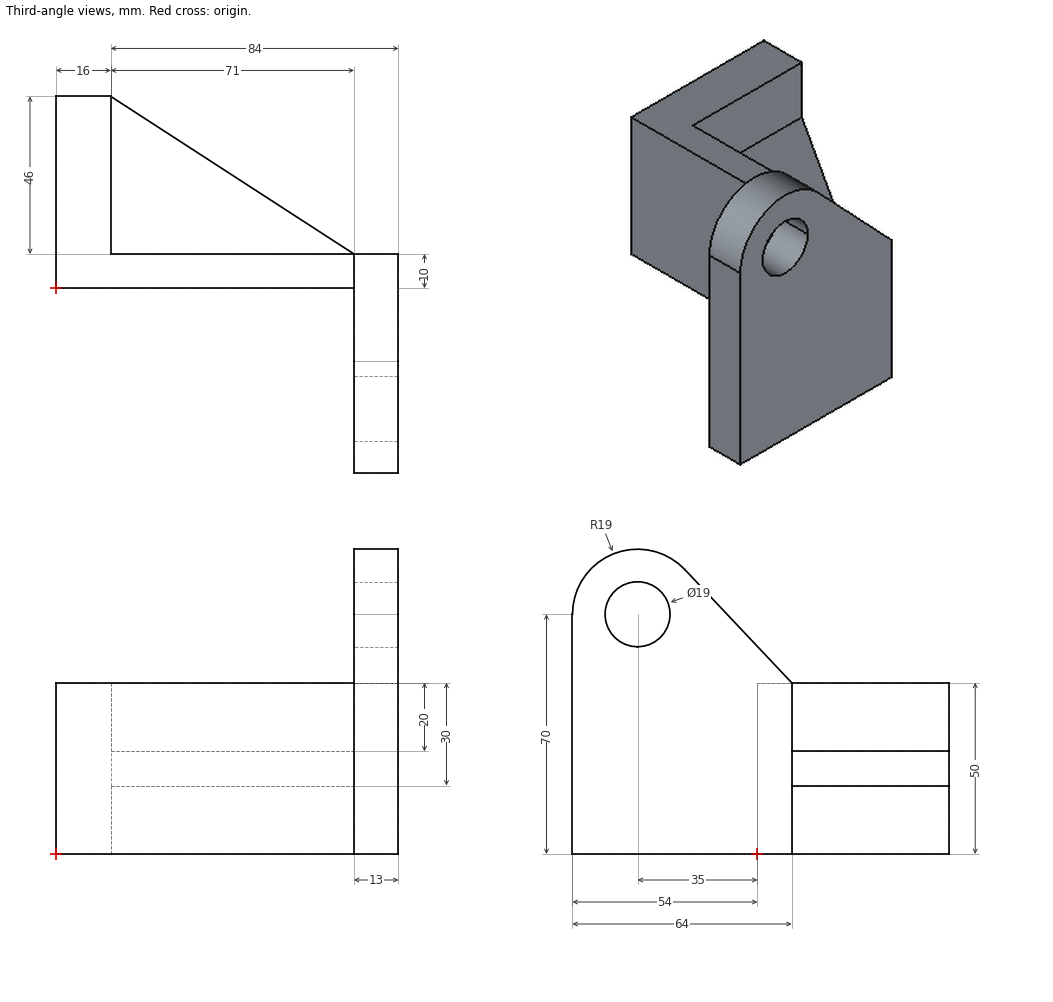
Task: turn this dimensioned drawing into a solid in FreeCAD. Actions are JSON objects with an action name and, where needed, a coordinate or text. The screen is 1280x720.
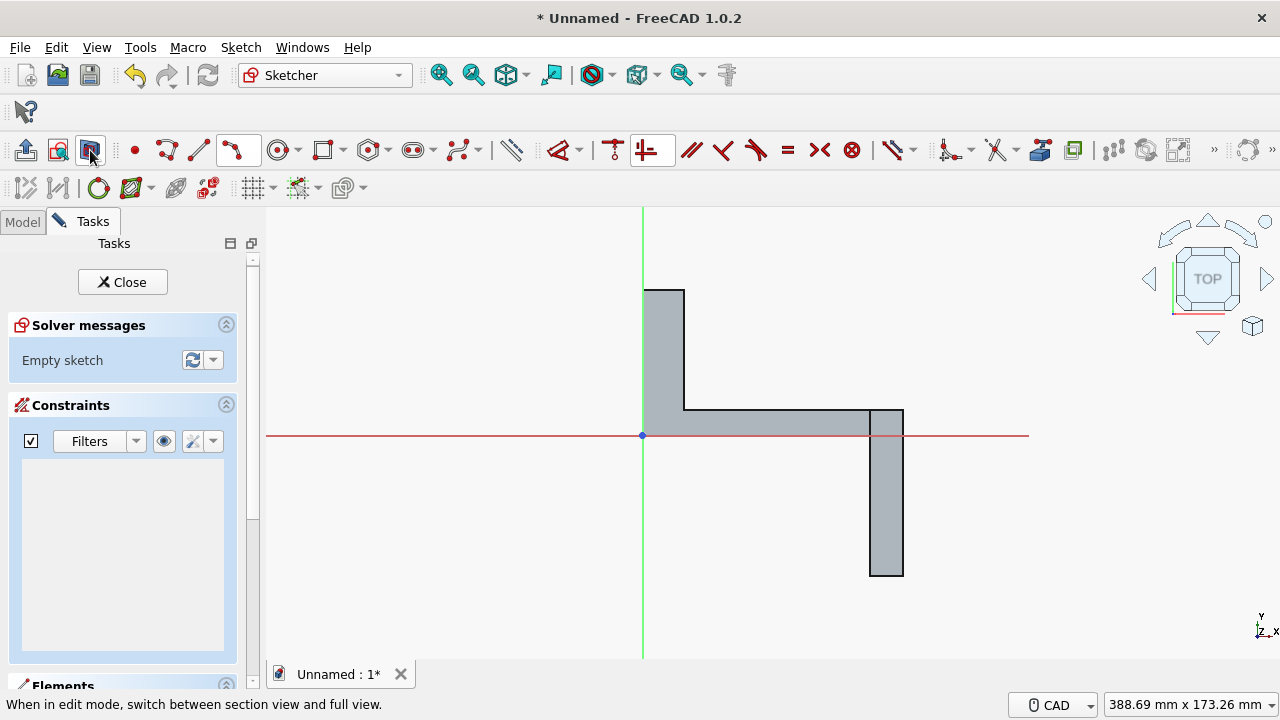
{"action": "scroll", "coordinate": [819, 277], "scroll_direction": "up", "scroll_amount": 3}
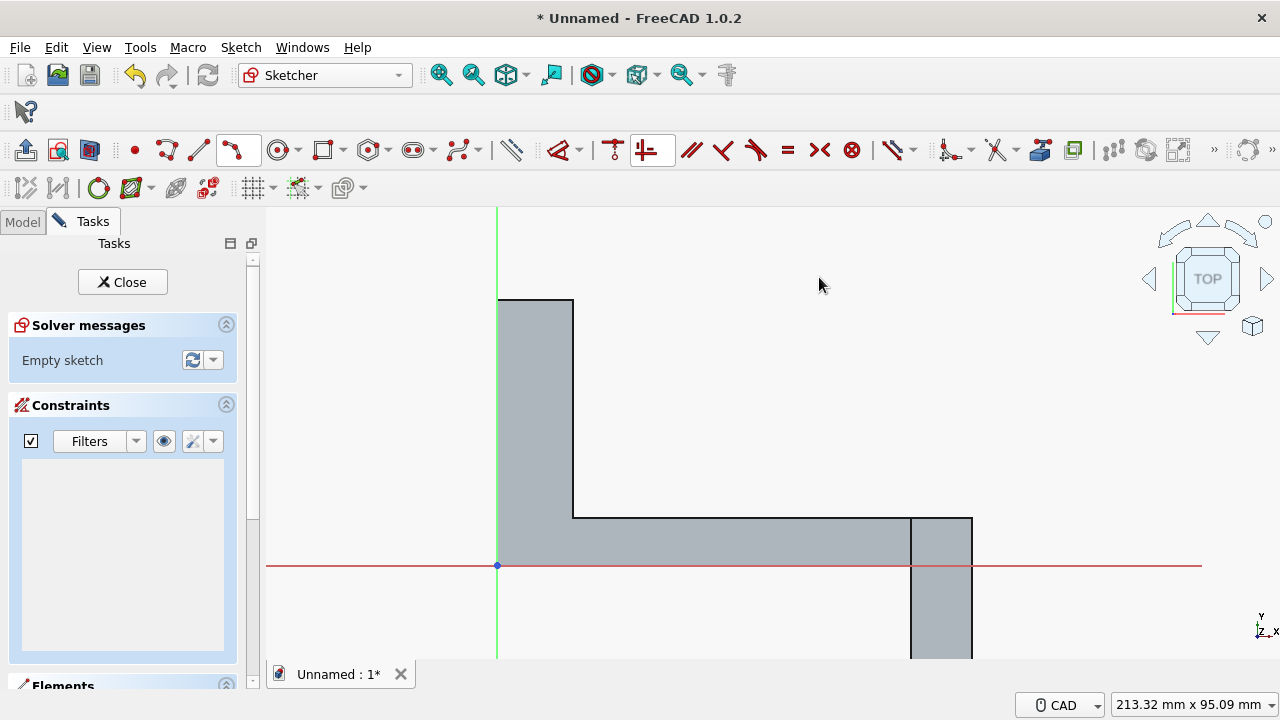
{"action": "left_click", "coordinate": [168, 150]}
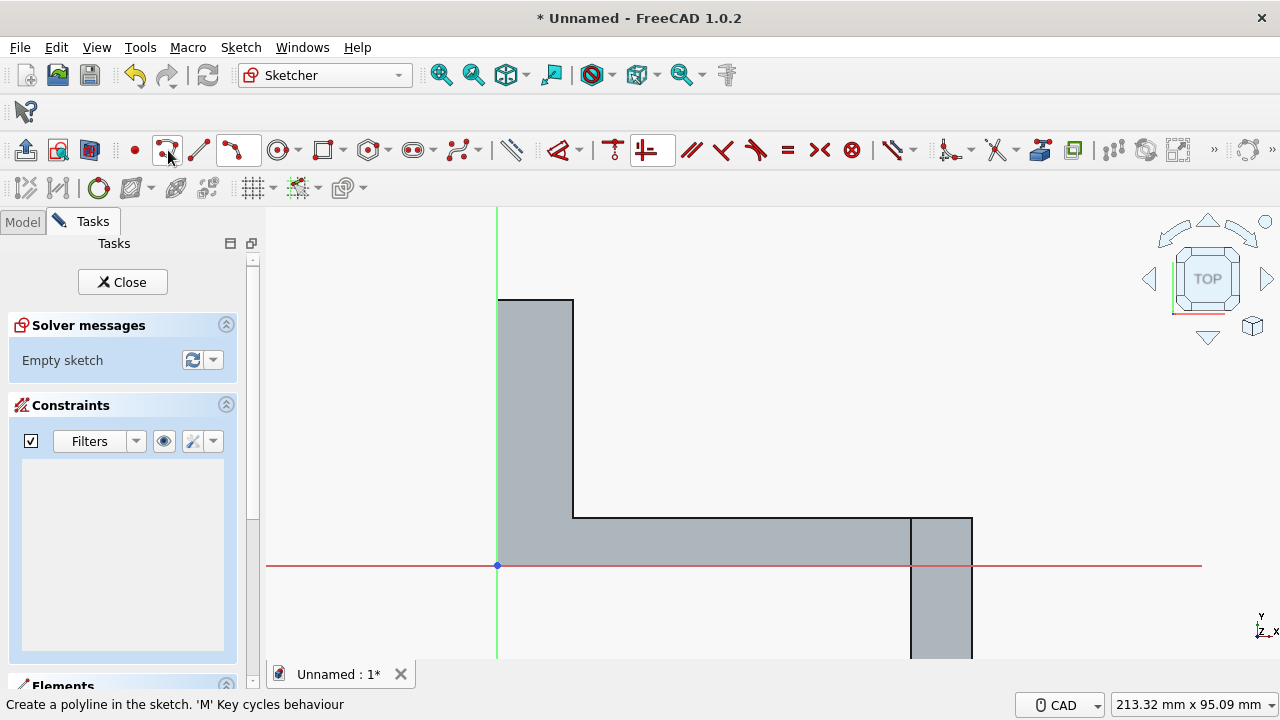
{"action": "left_click", "coordinate": [573, 518]}
{"action": "left_click", "coordinate": [911, 518]}
{"action": "left_click", "coordinate": [573, 300]}
{"action": "left_click", "coordinate": [573, 519]}
{"action": "key", "text": "Escape"}
{"action": "key", "text": "Escape"}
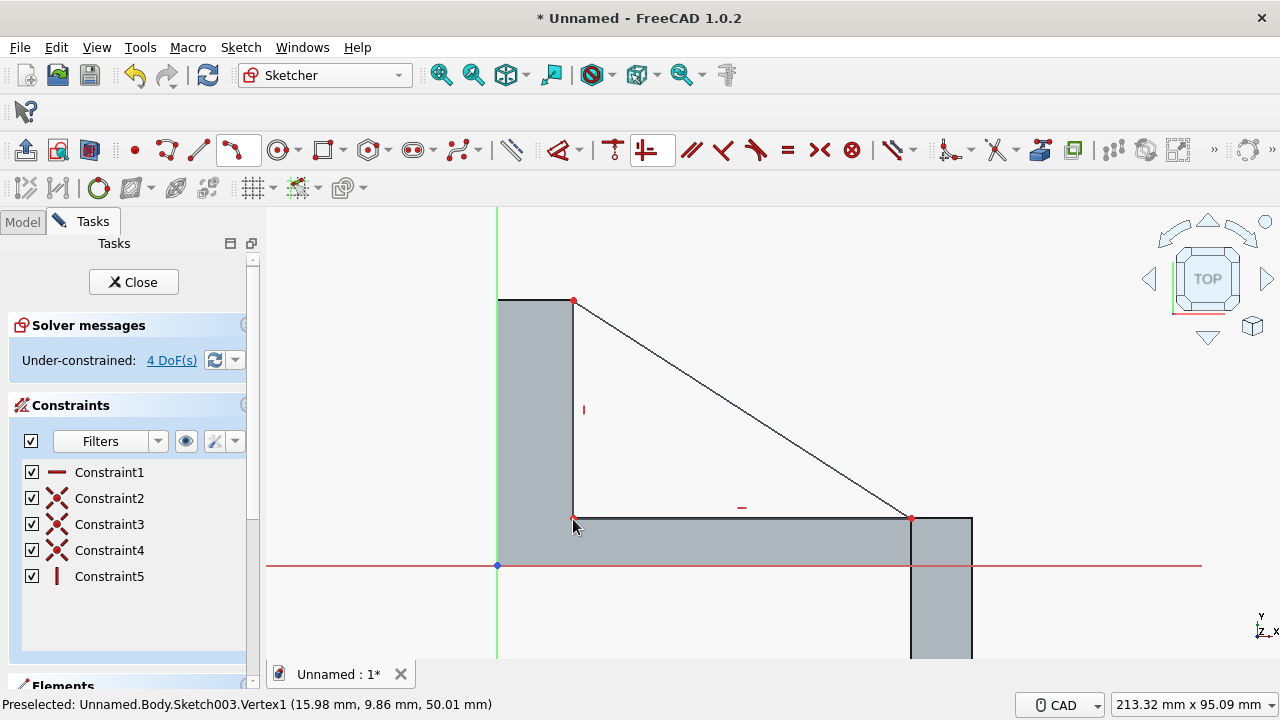
{"action": "key", "text": "d"}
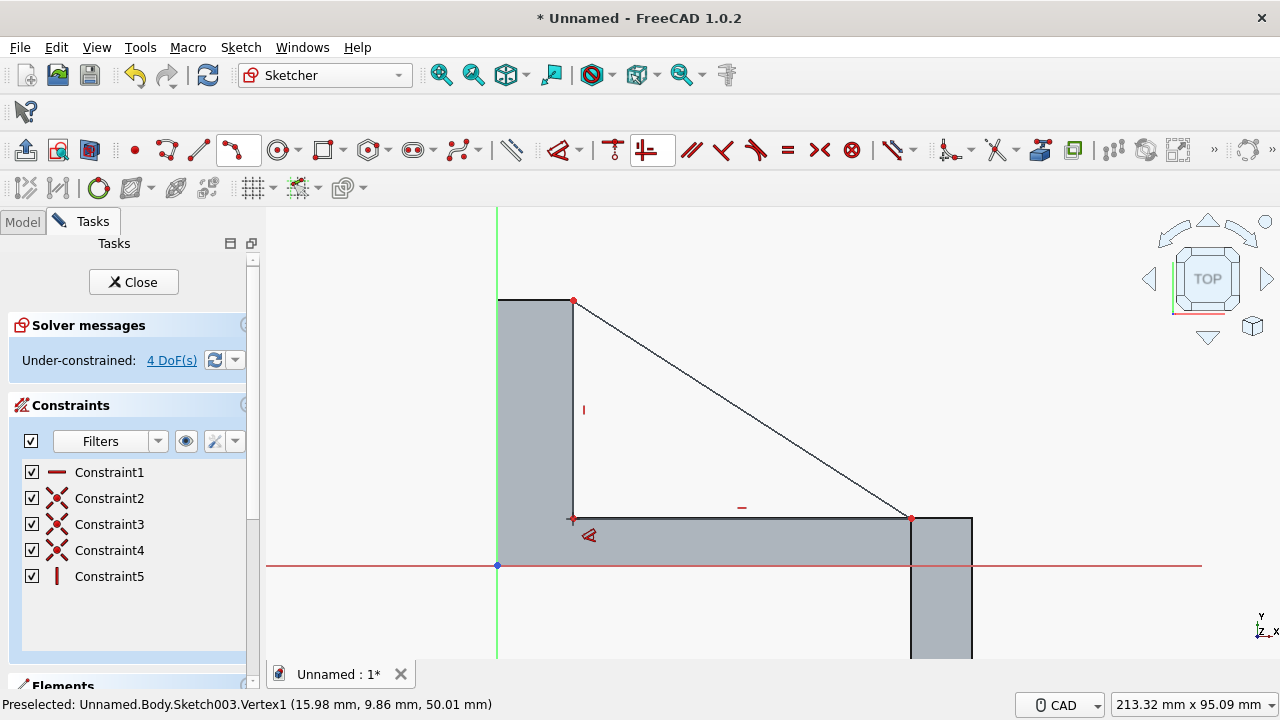
{"action": "left_click", "coordinate": [674, 519]}
{"action": "left_click", "coordinate": [742, 485]}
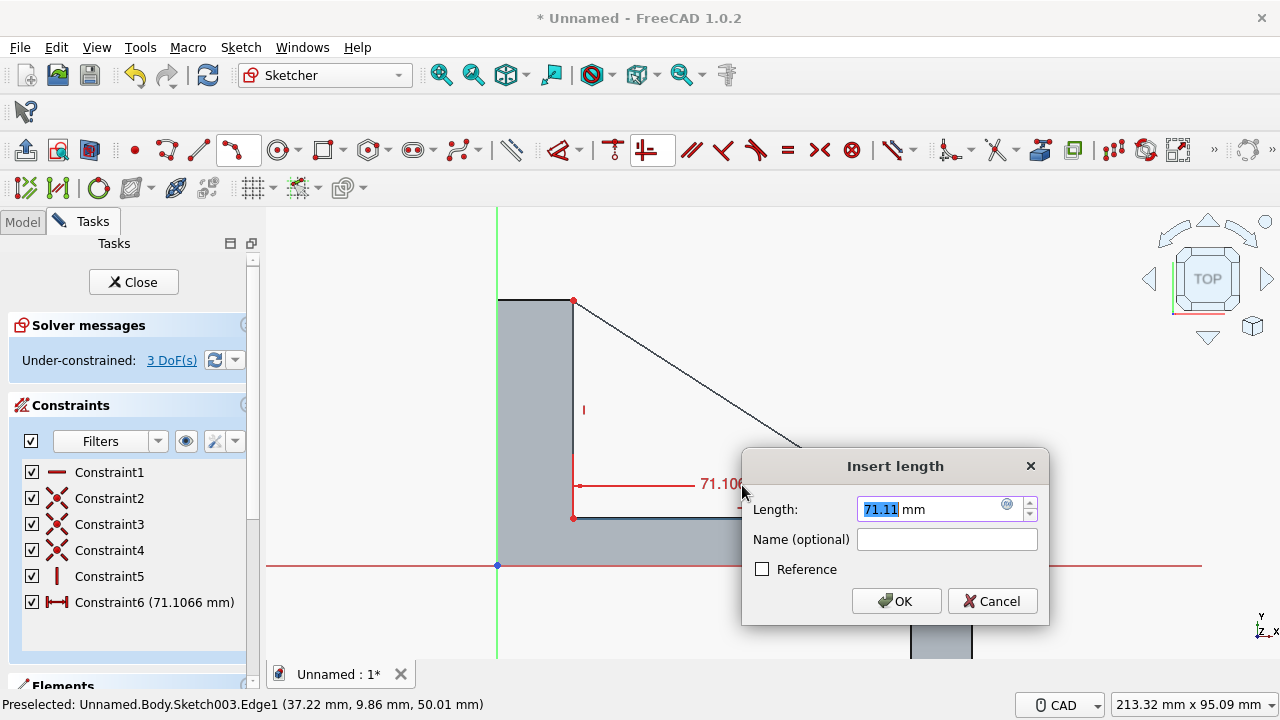
{"action": "type", "text": "71"}
{"action": "key", "text": "Return"}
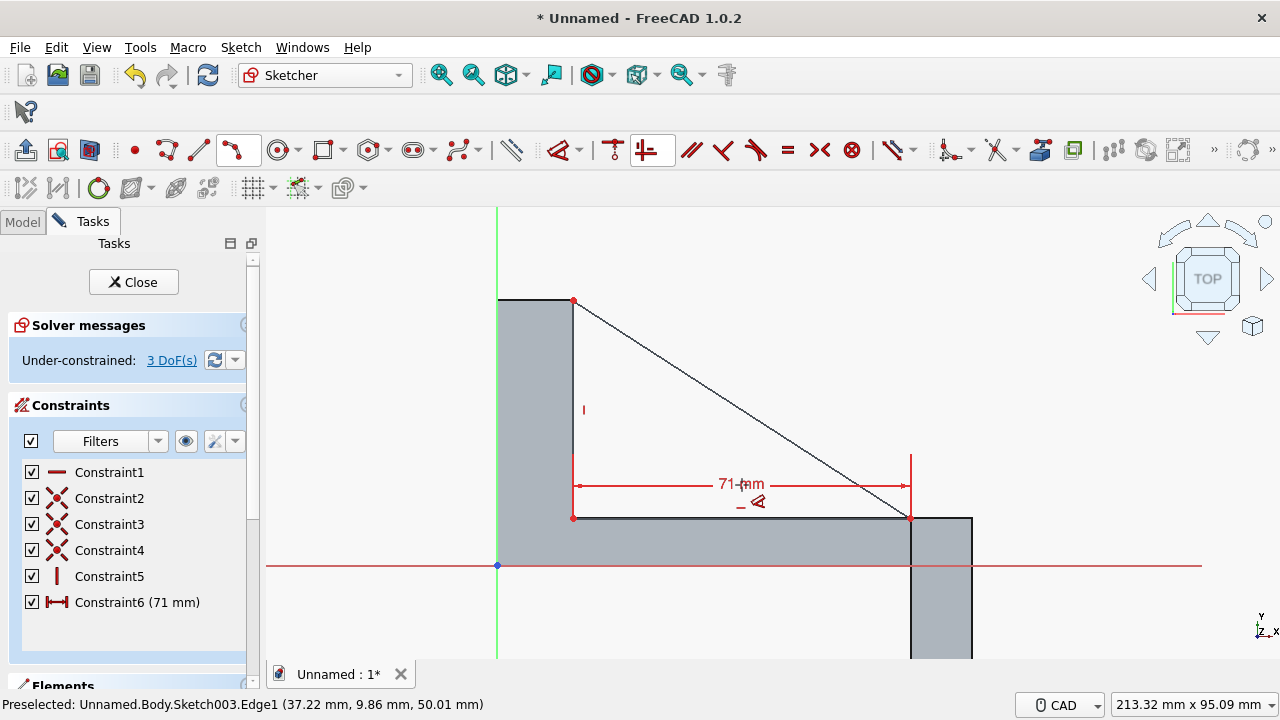
{"action": "left_click", "coordinate": [573, 366]}
{"action": "left_click", "coordinate": [539, 410]}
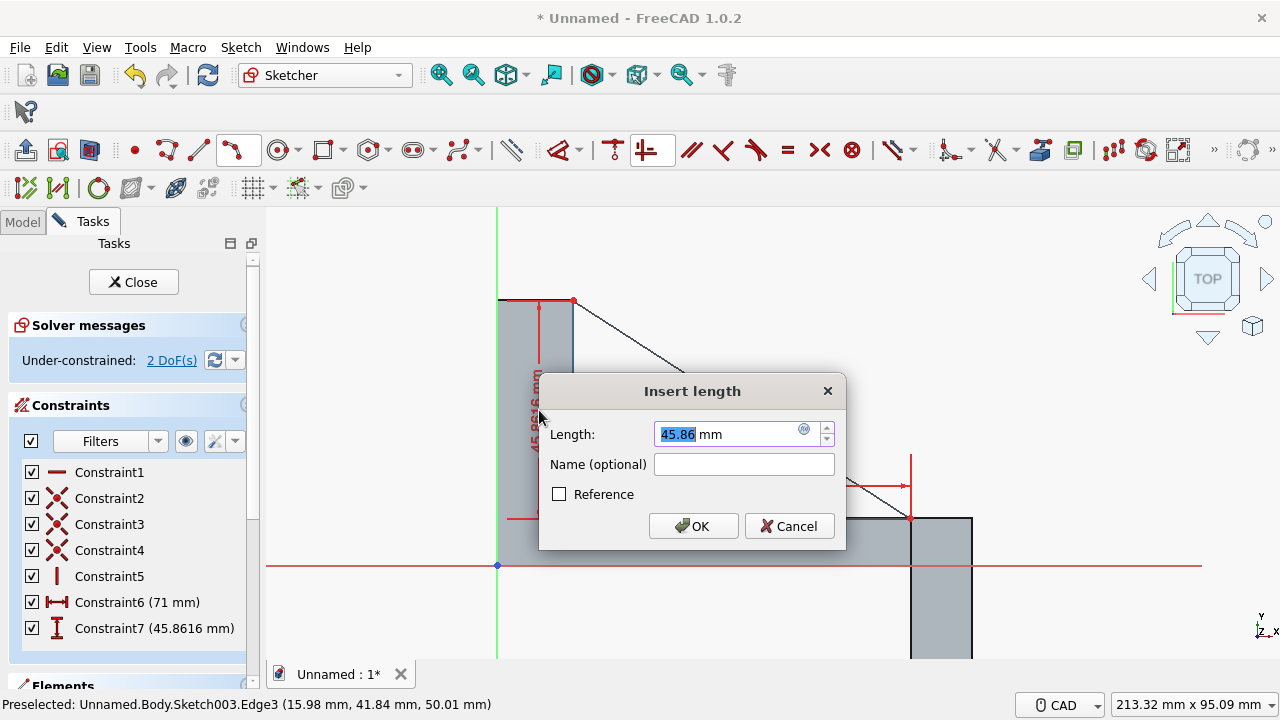
{"action": "type", "text": "46"}
{"action": "key", "text": "Return"}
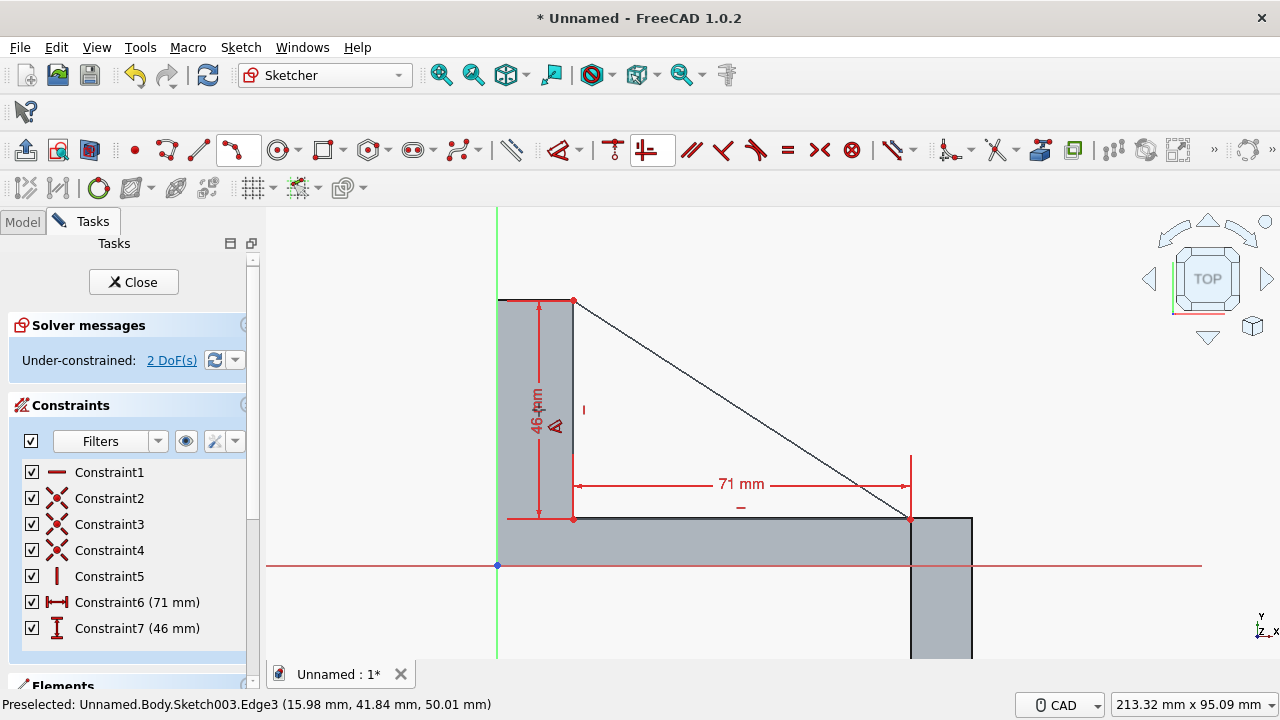
{"action": "left_click", "coordinate": [573, 519]}
{"action": "left_click", "coordinate": [535, 600]}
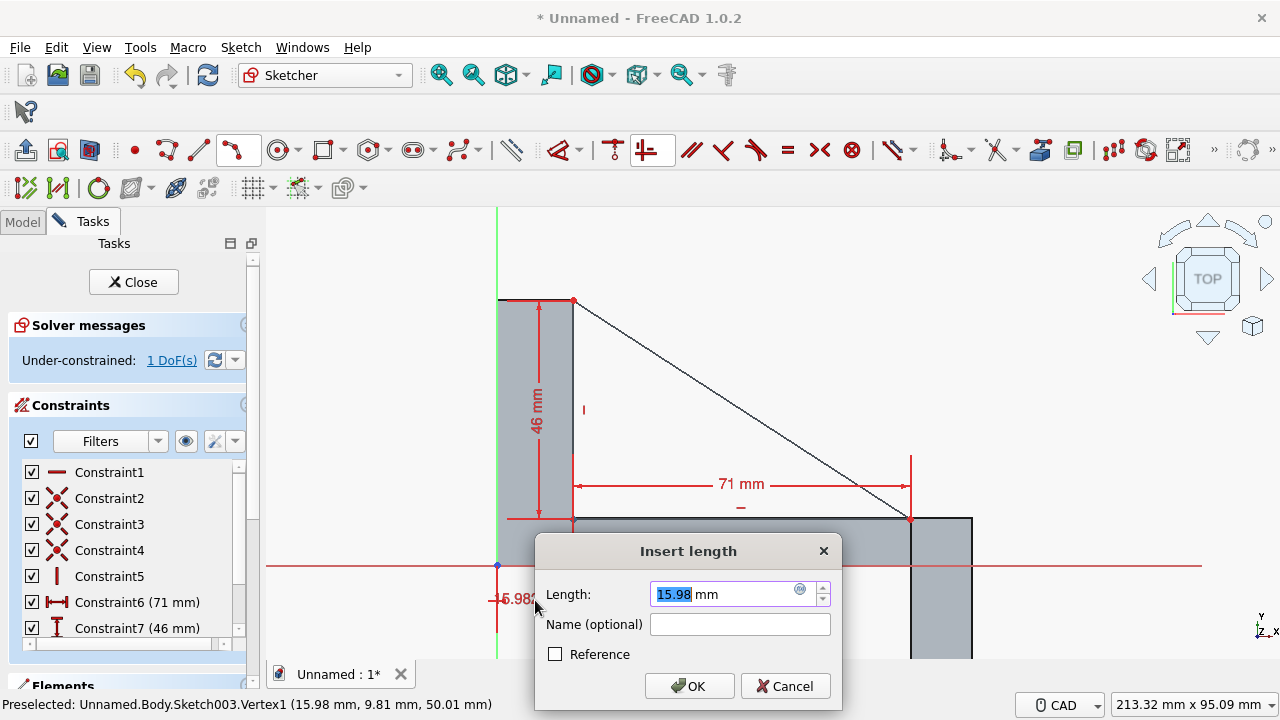
{"action": "type", "text": "16"}
{"action": "key", "text": "Return"}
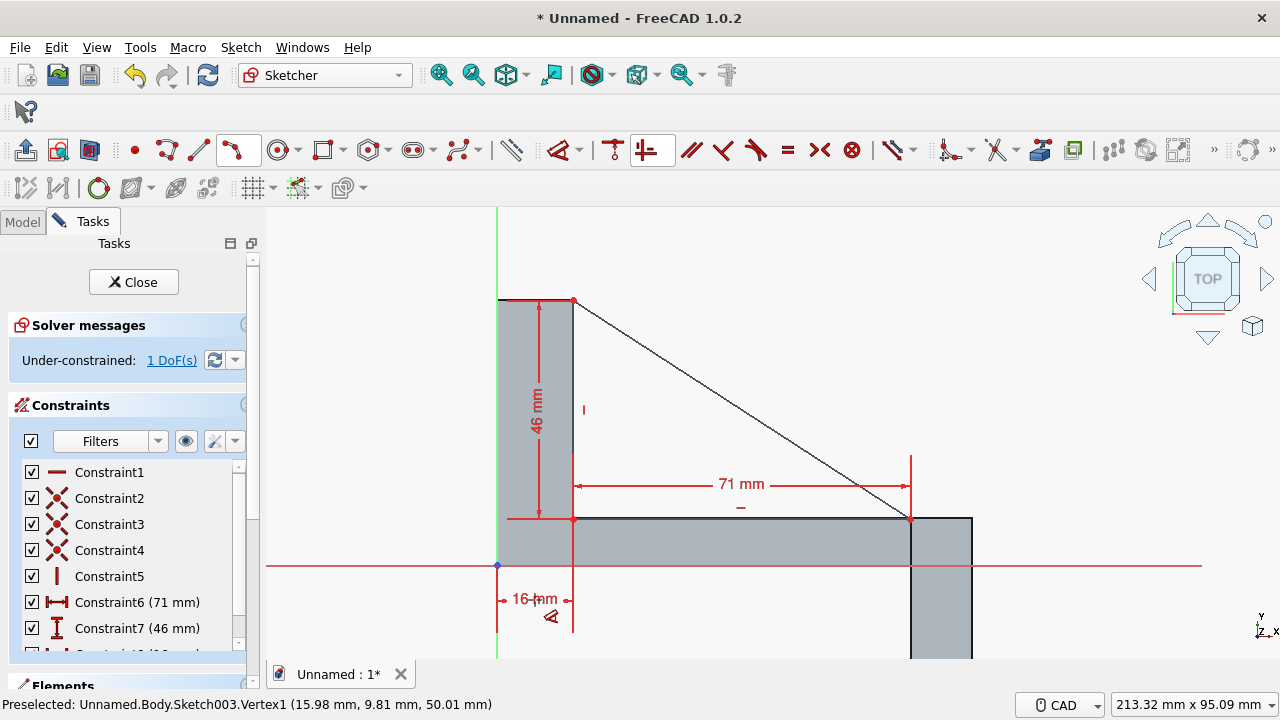
{"action": "left_click", "coordinate": [573, 519]}
{"action": "left_click", "coordinate": [463, 543]}